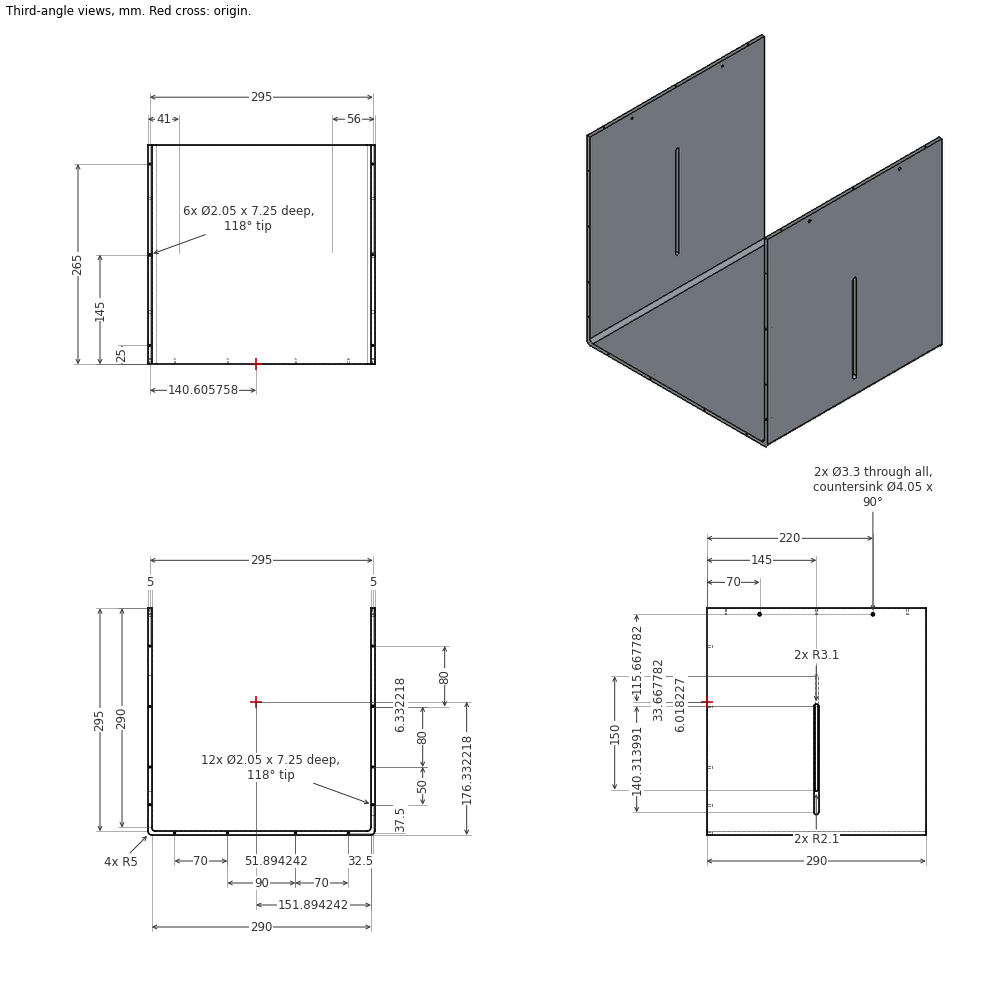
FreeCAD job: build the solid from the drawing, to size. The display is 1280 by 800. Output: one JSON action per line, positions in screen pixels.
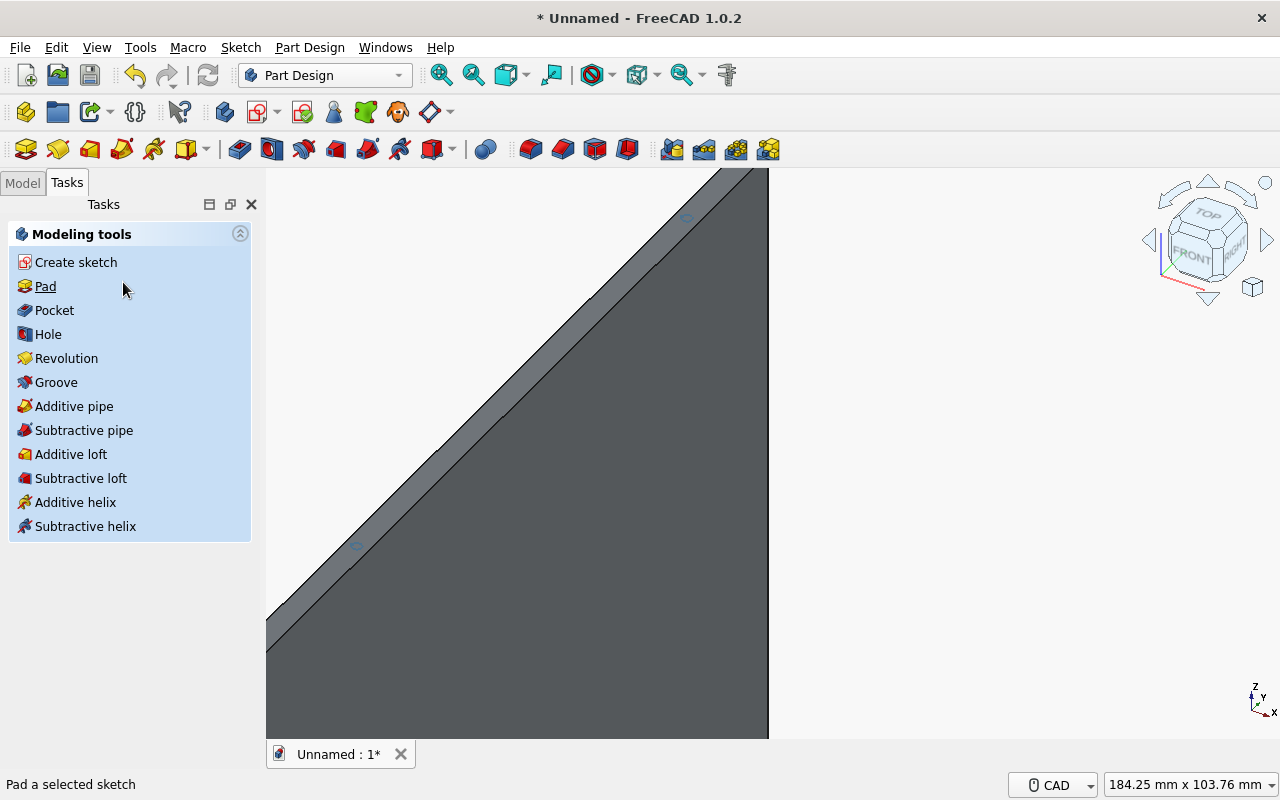
{"action": "left_click", "coordinate": [272, 150]}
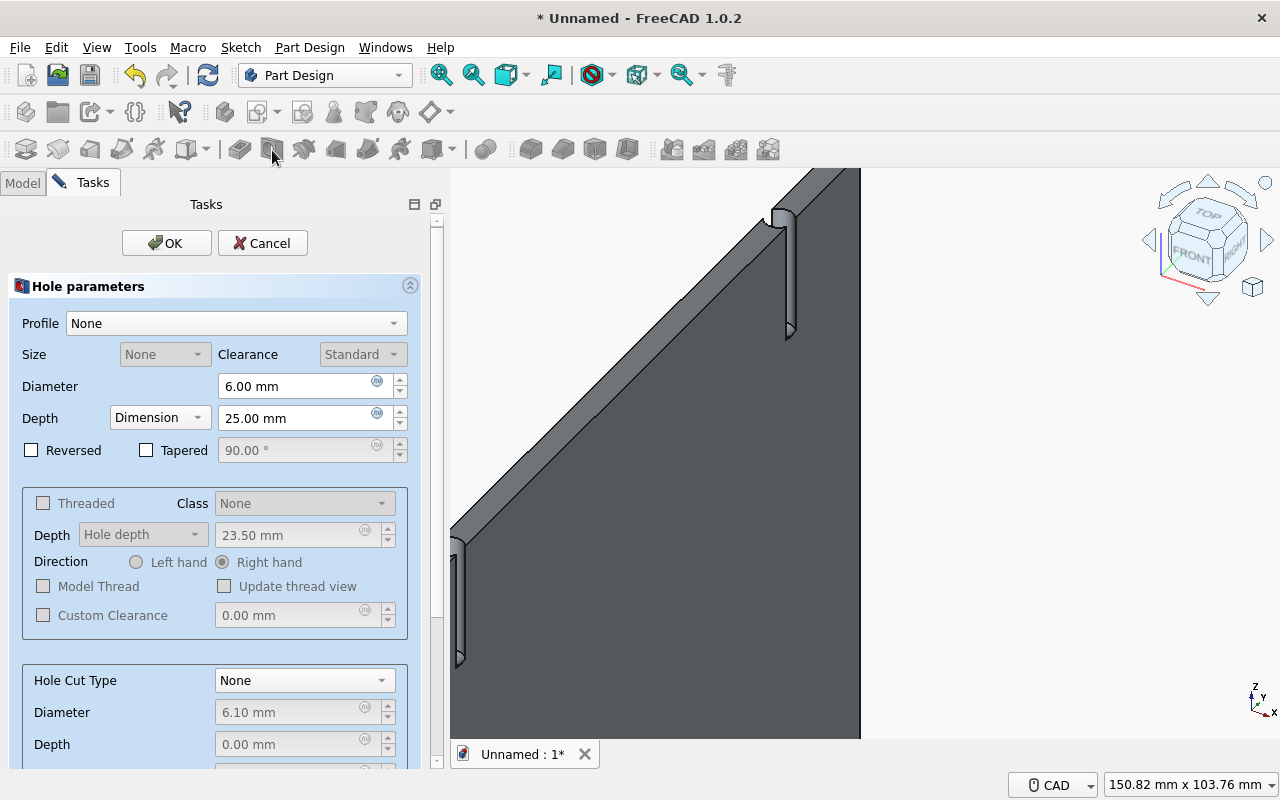
{"action": "triple_click", "coordinate": [305, 386]}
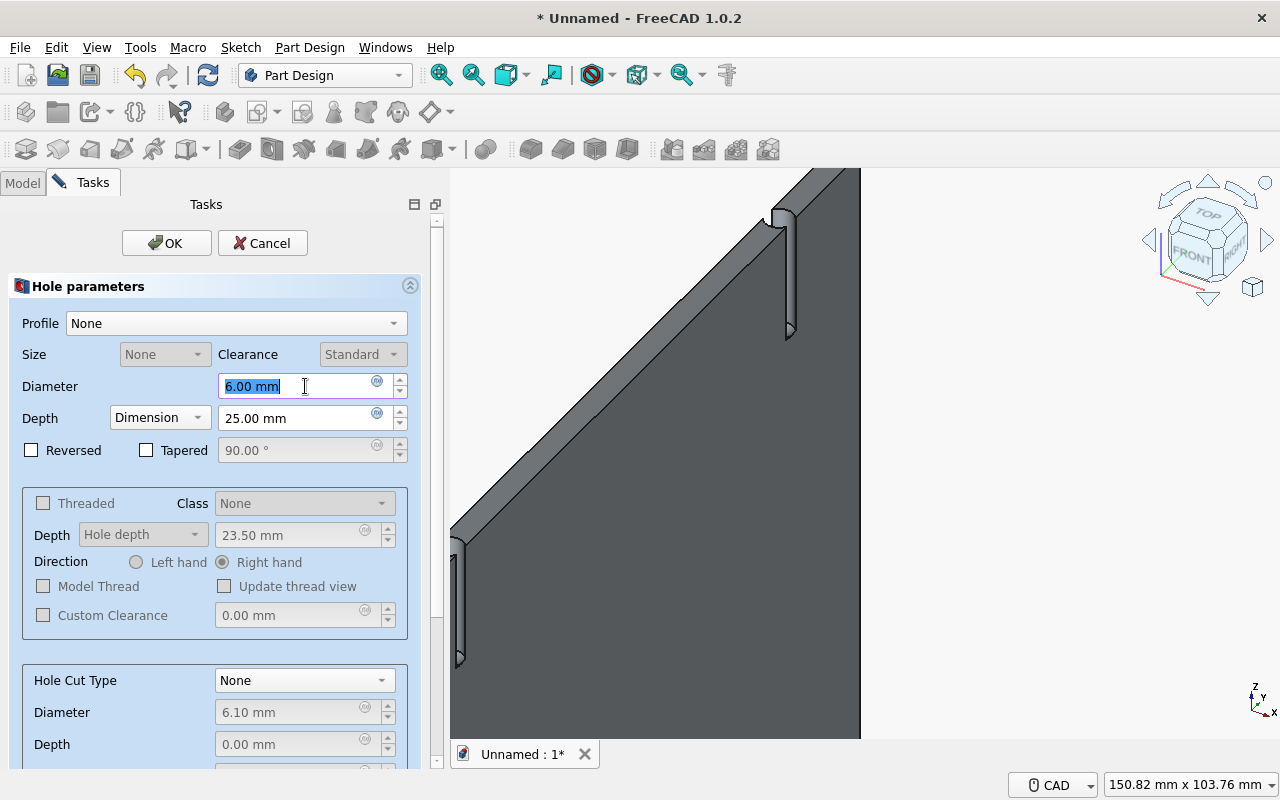
{"action": "type", "text": "2.05"}
{"action": "key", "text": "Tab"}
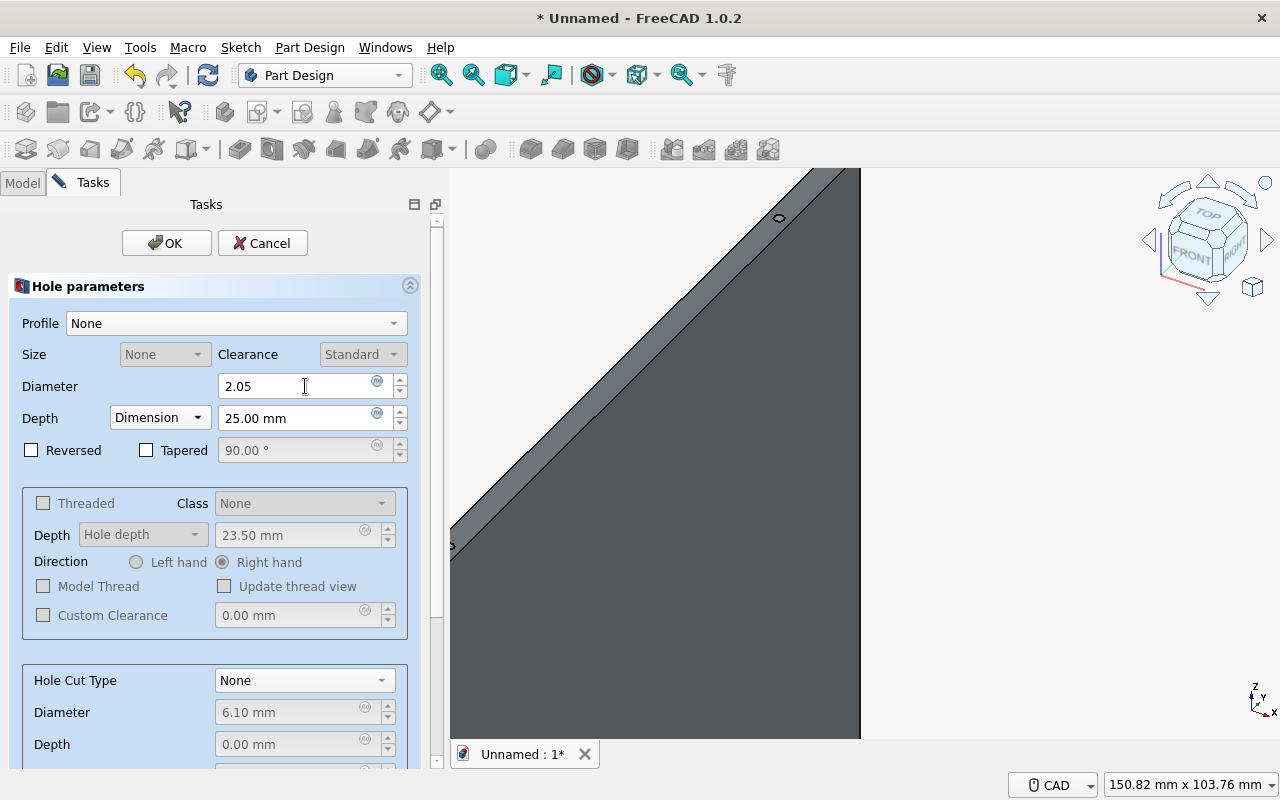
{"action": "triple_click", "coordinate": [305, 418]}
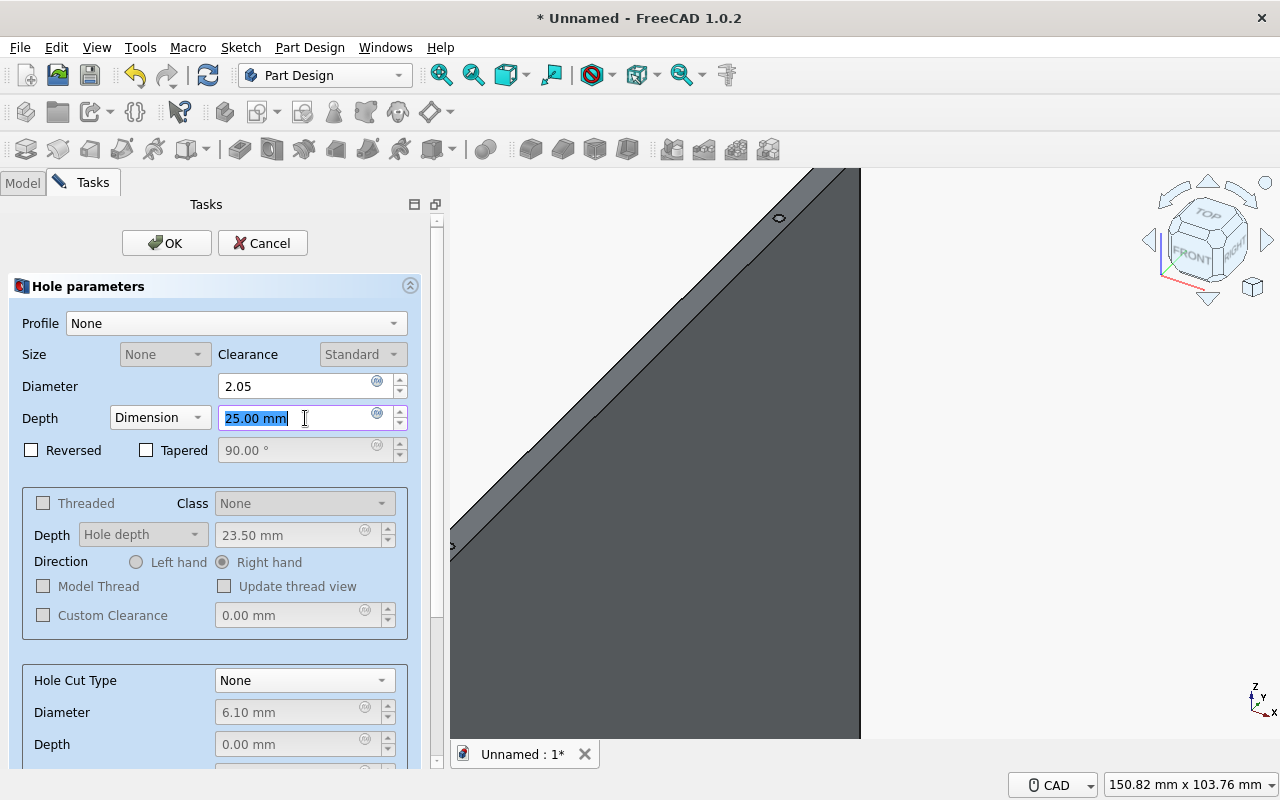
{"action": "type", "text": "7.25"}
{"action": "key", "text": "Tab"}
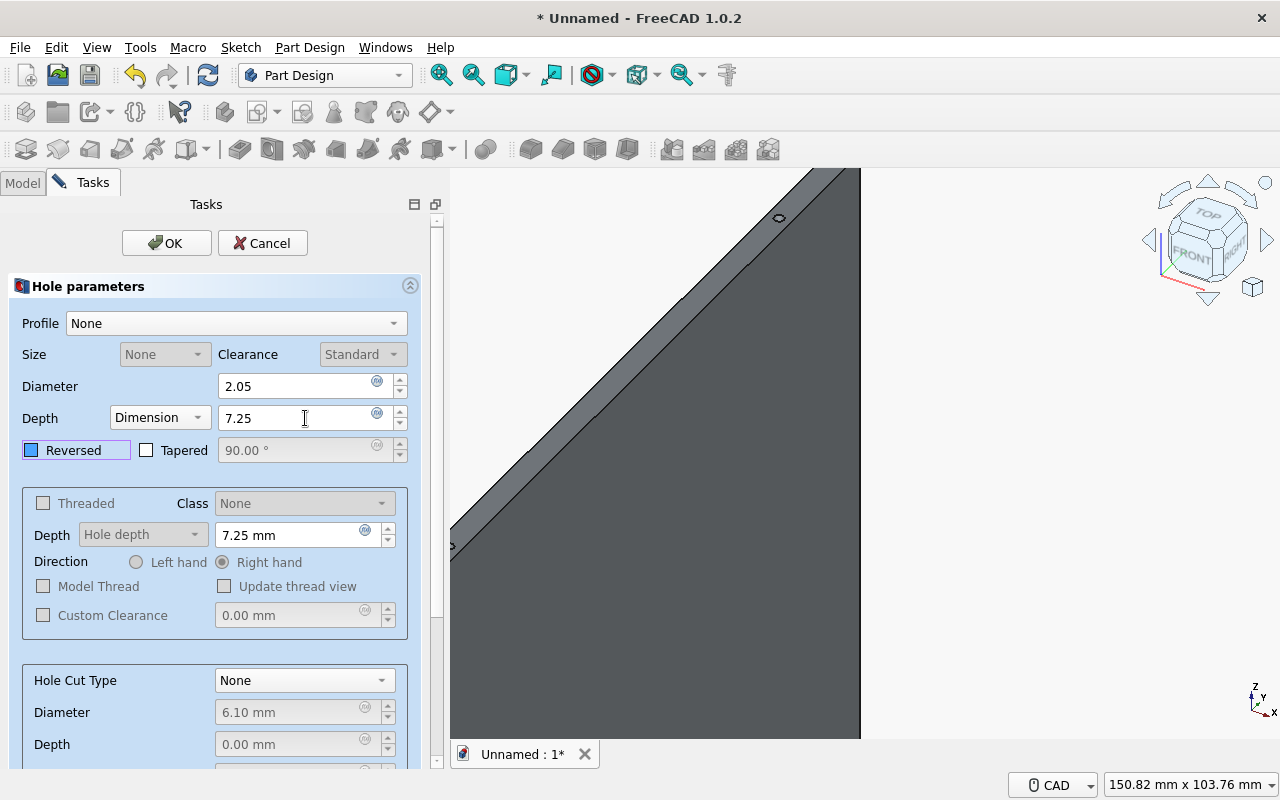
{"action": "left_click", "coordinate": [167, 243]}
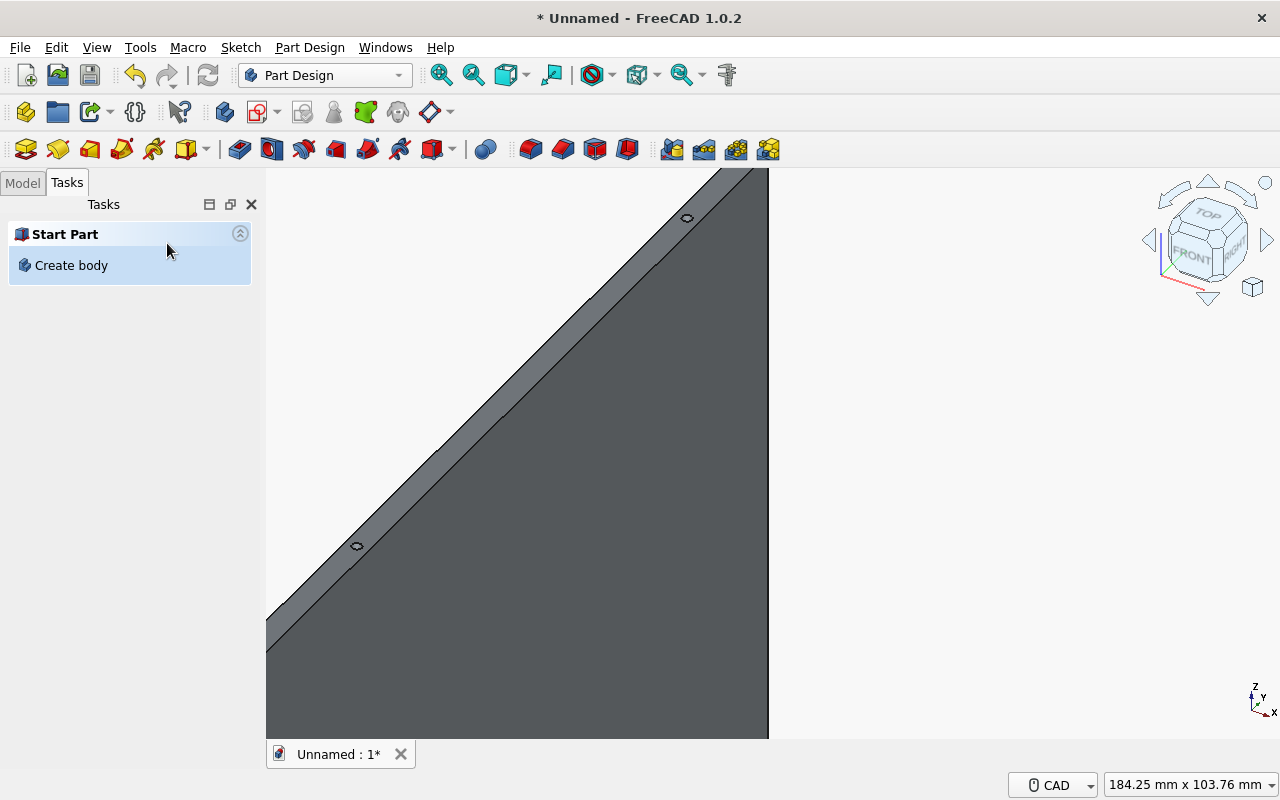
{"action": "left_click", "coordinate": [442, 76]}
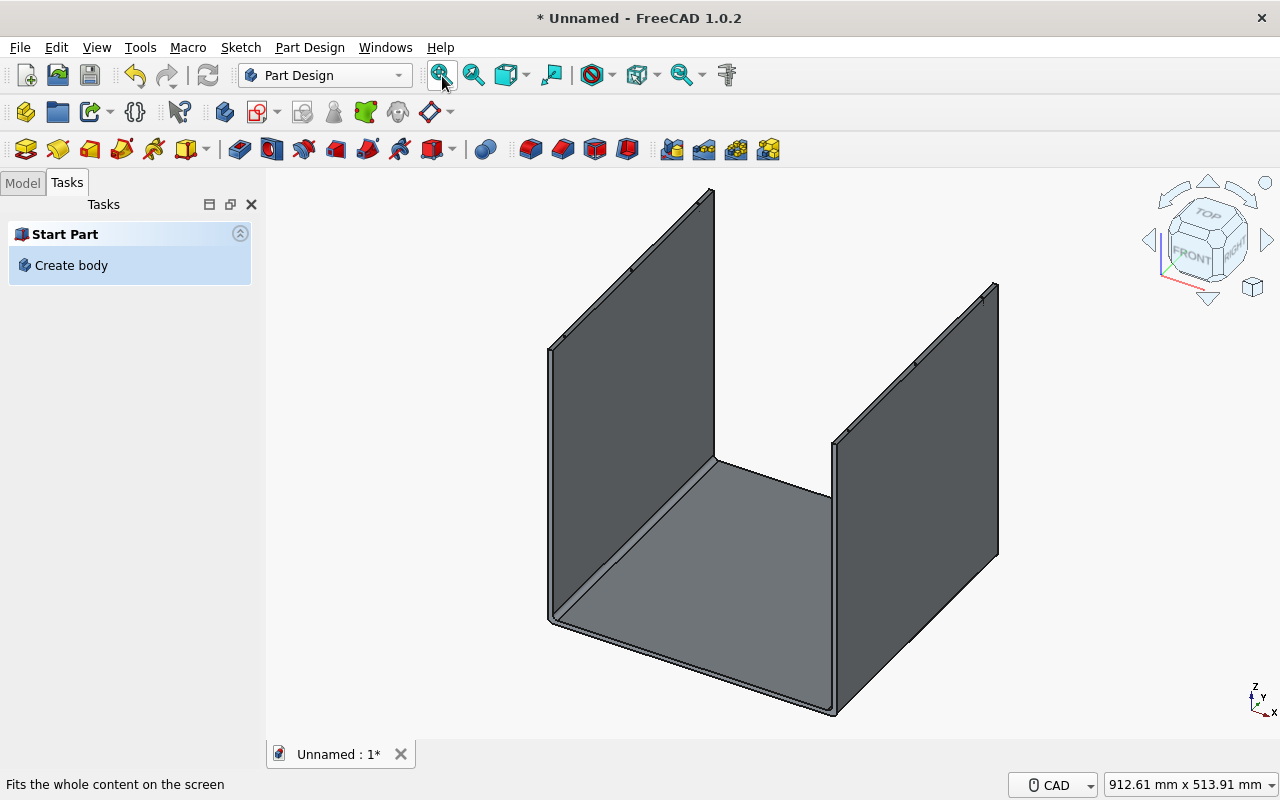
{"action": "key", "text": "6"}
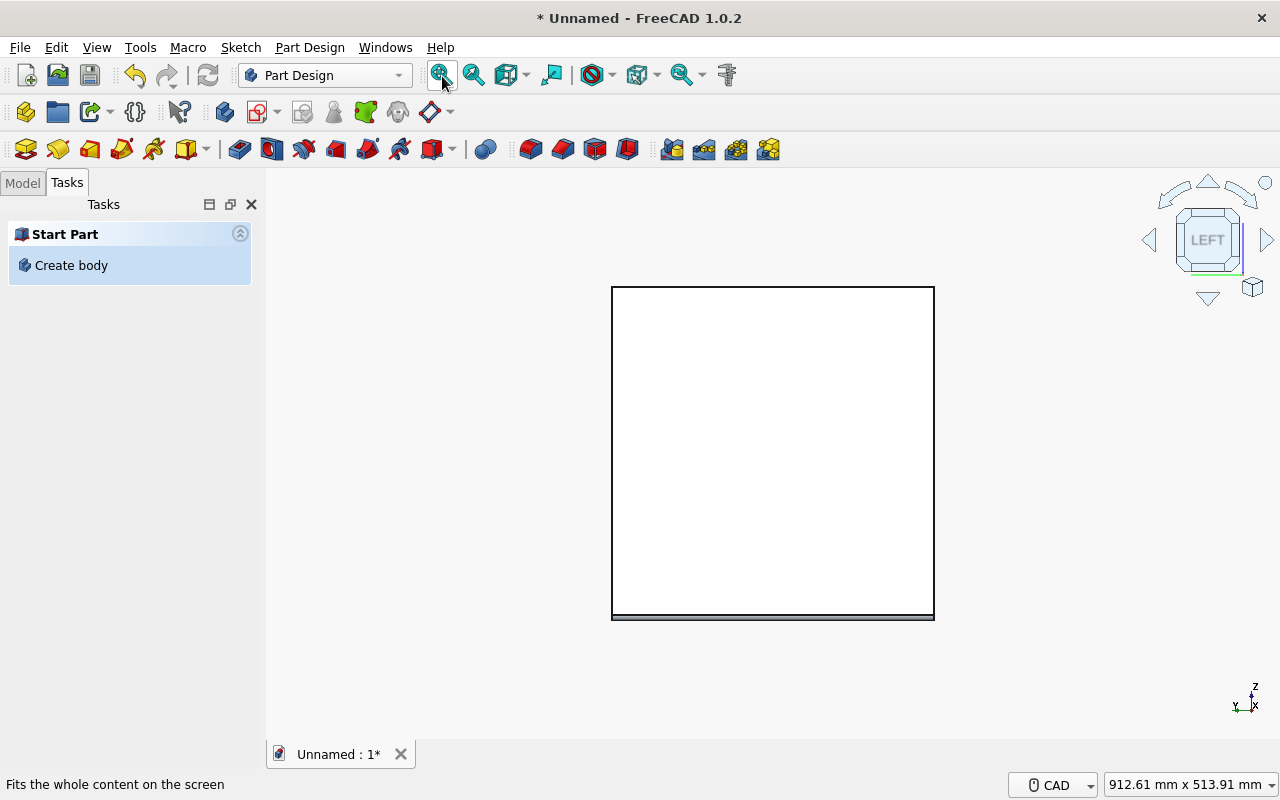
{"action": "left_click", "coordinate": [773, 450]}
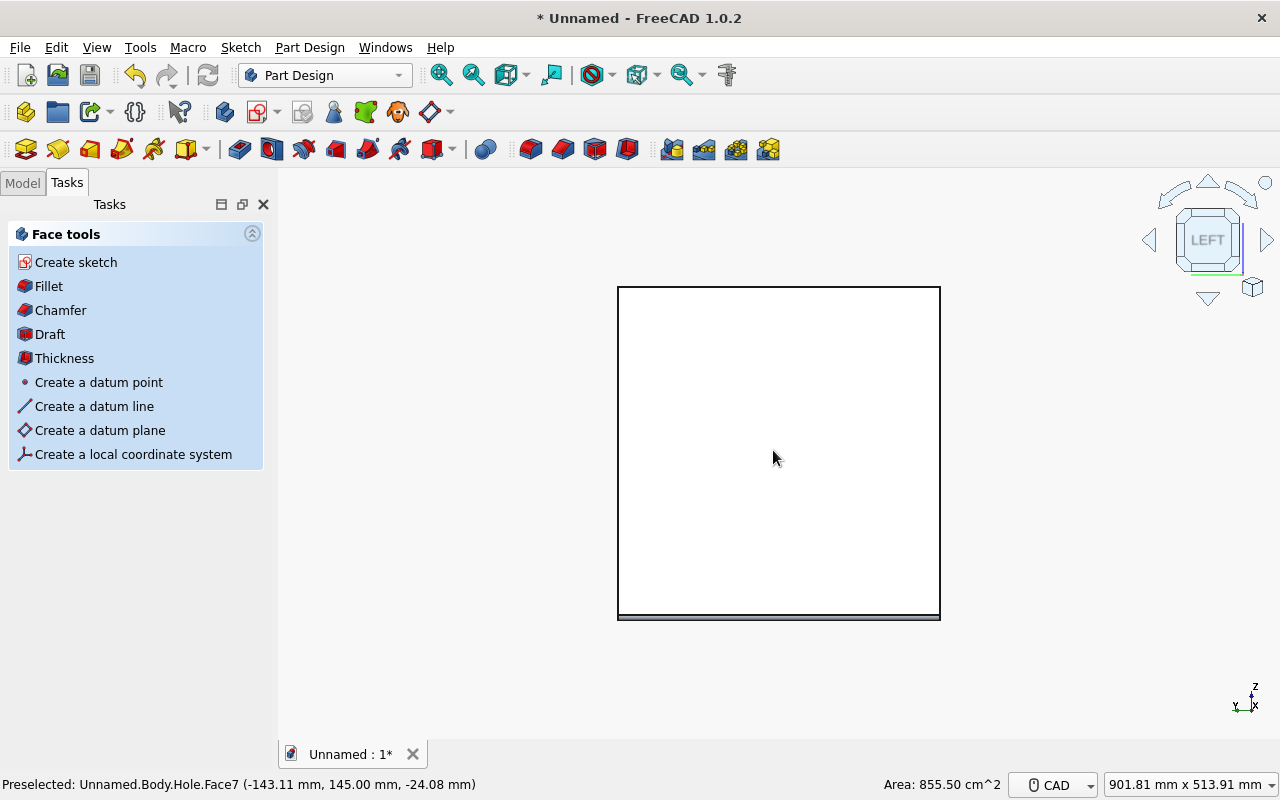
{"action": "left_click", "coordinate": [258, 112]}